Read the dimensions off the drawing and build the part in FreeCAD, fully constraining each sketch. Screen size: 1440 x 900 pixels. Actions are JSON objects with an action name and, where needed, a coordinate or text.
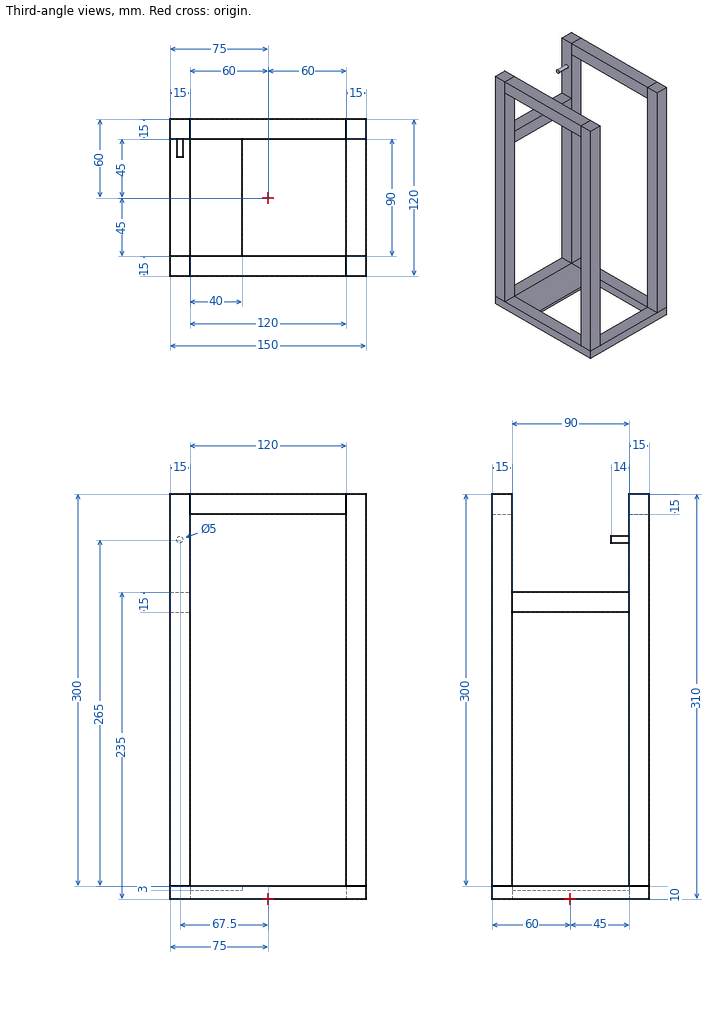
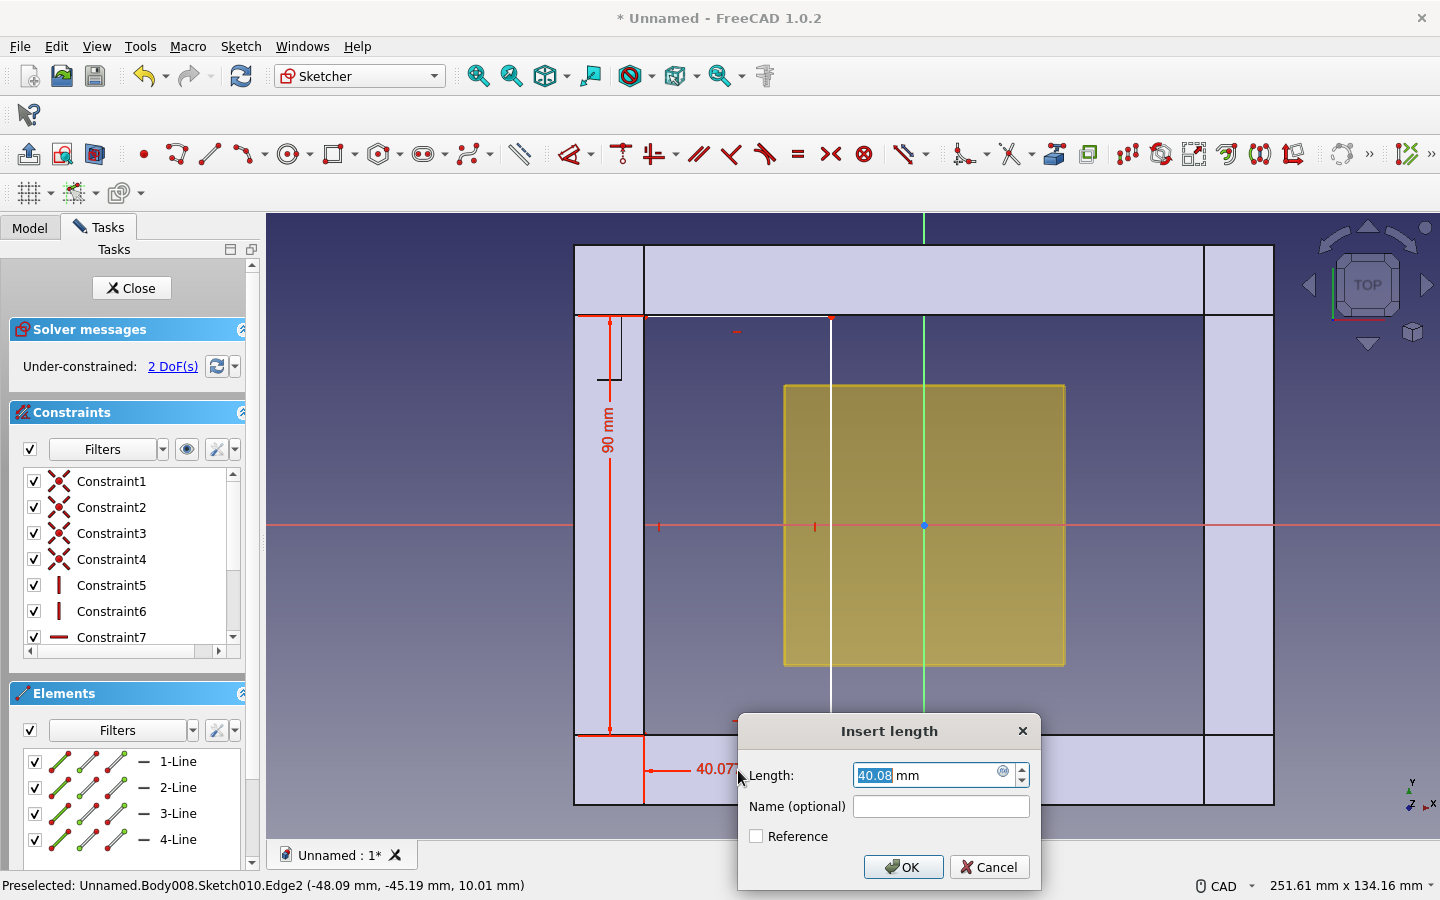
{"action": "type", "text": "40"}
{"action": "key", "text": "Return"}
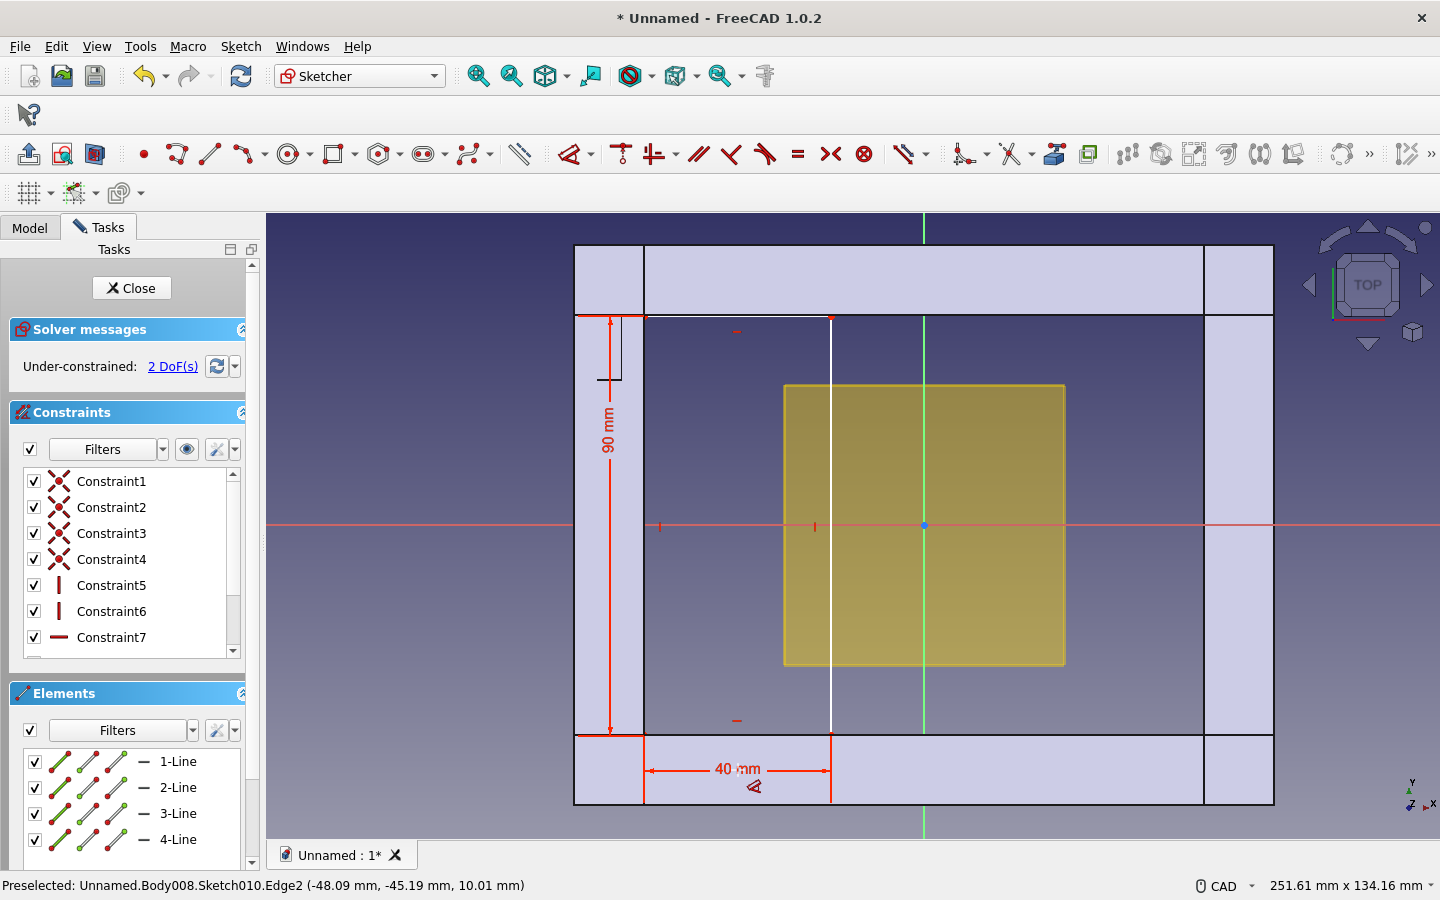
{"action": "left_click", "coordinate": [644, 316]}
{"action": "left_click", "coordinate": [784, 282]}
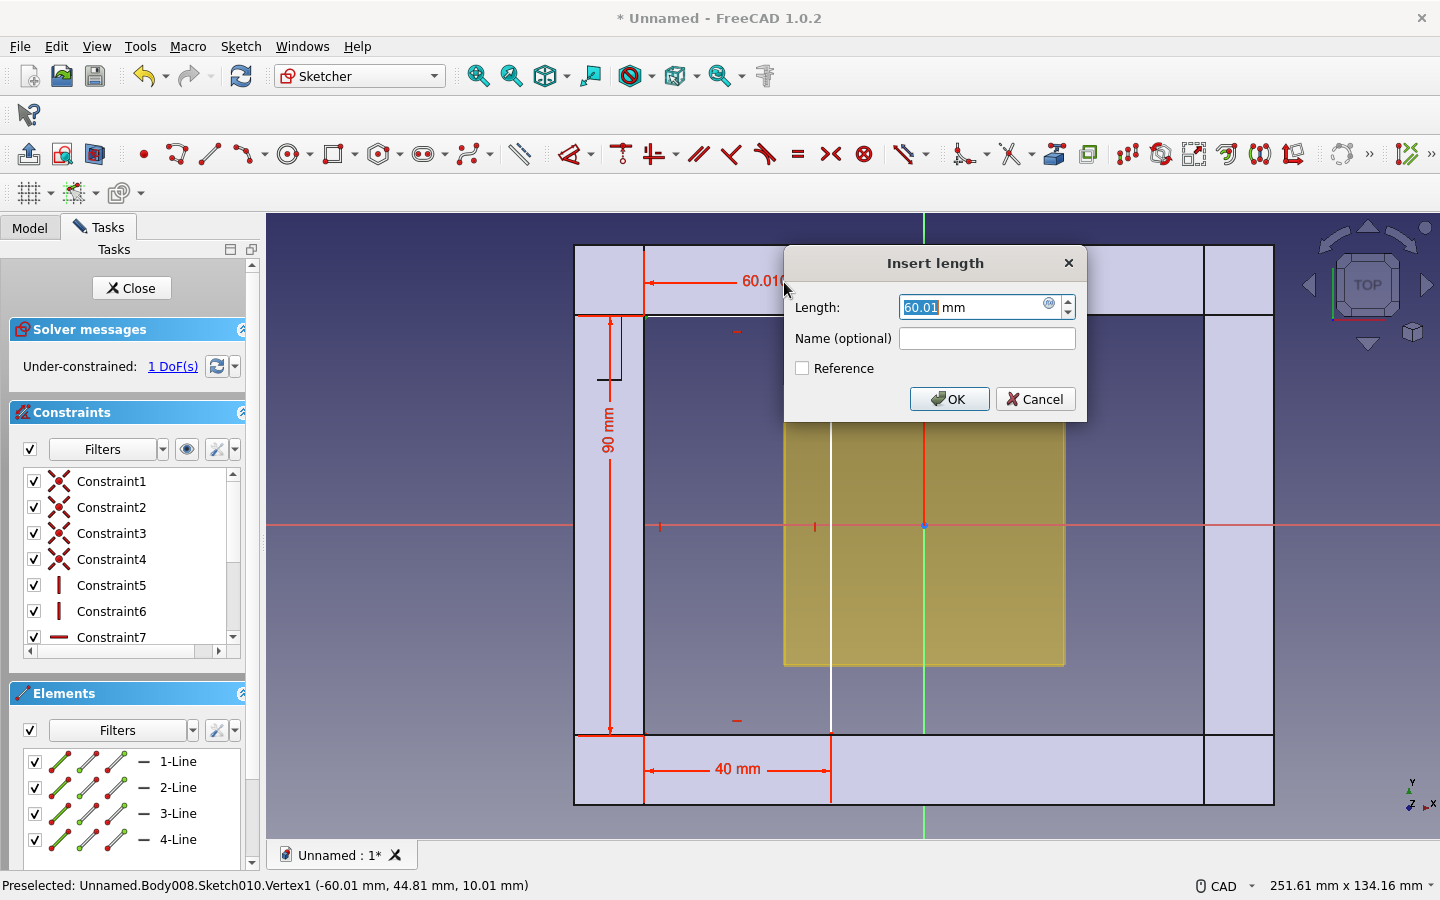
{"action": "type", "text": "60"}
{"action": "key", "text": "Return"}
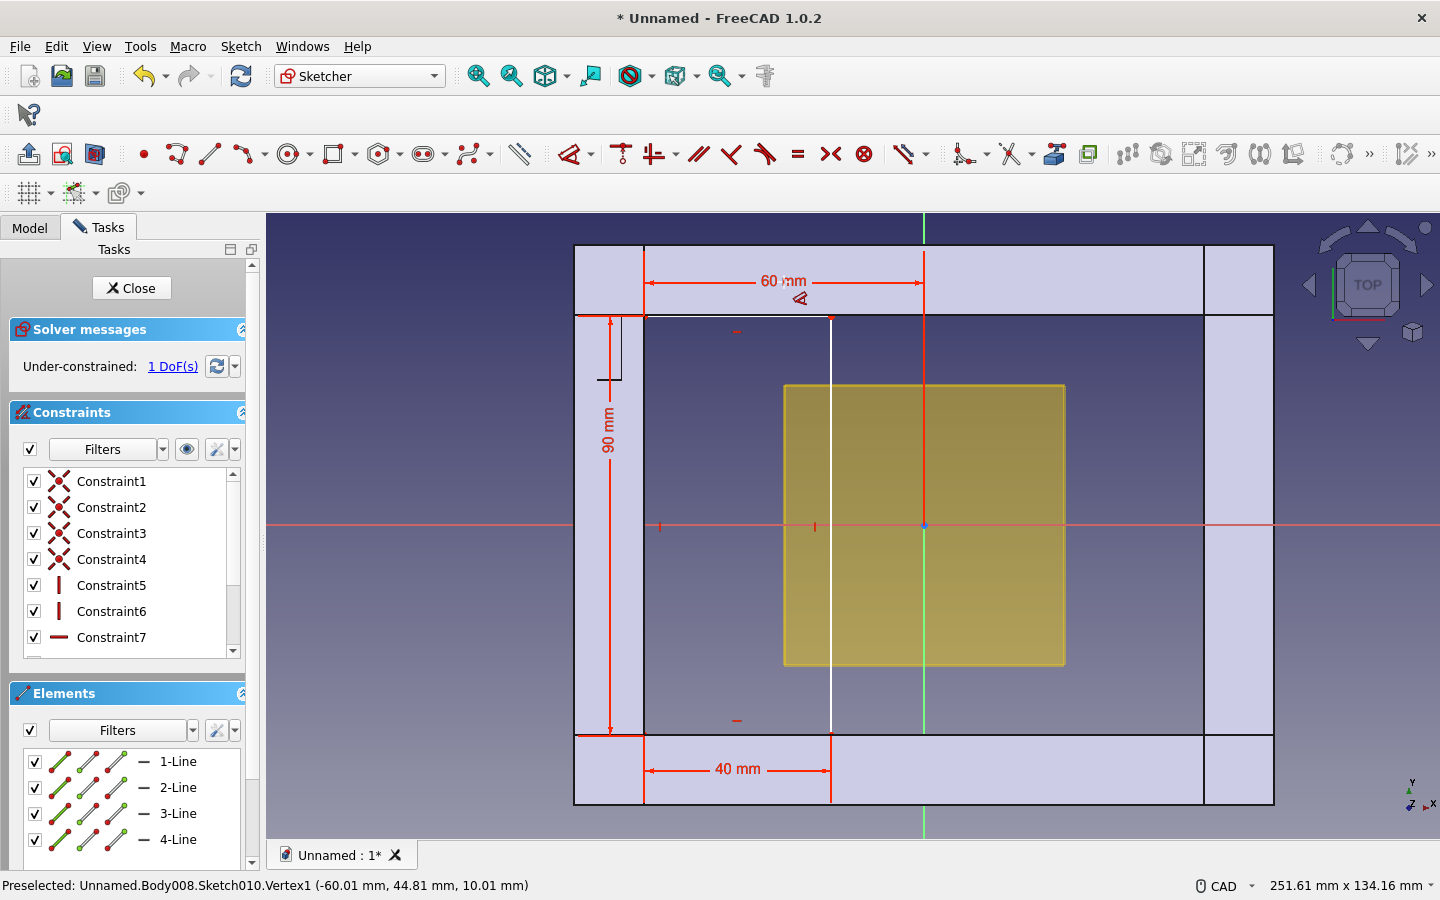
{"action": "left_click", "coordinate": [644, 316]}
{"action": "left_click", "coordinate": [958, 421]}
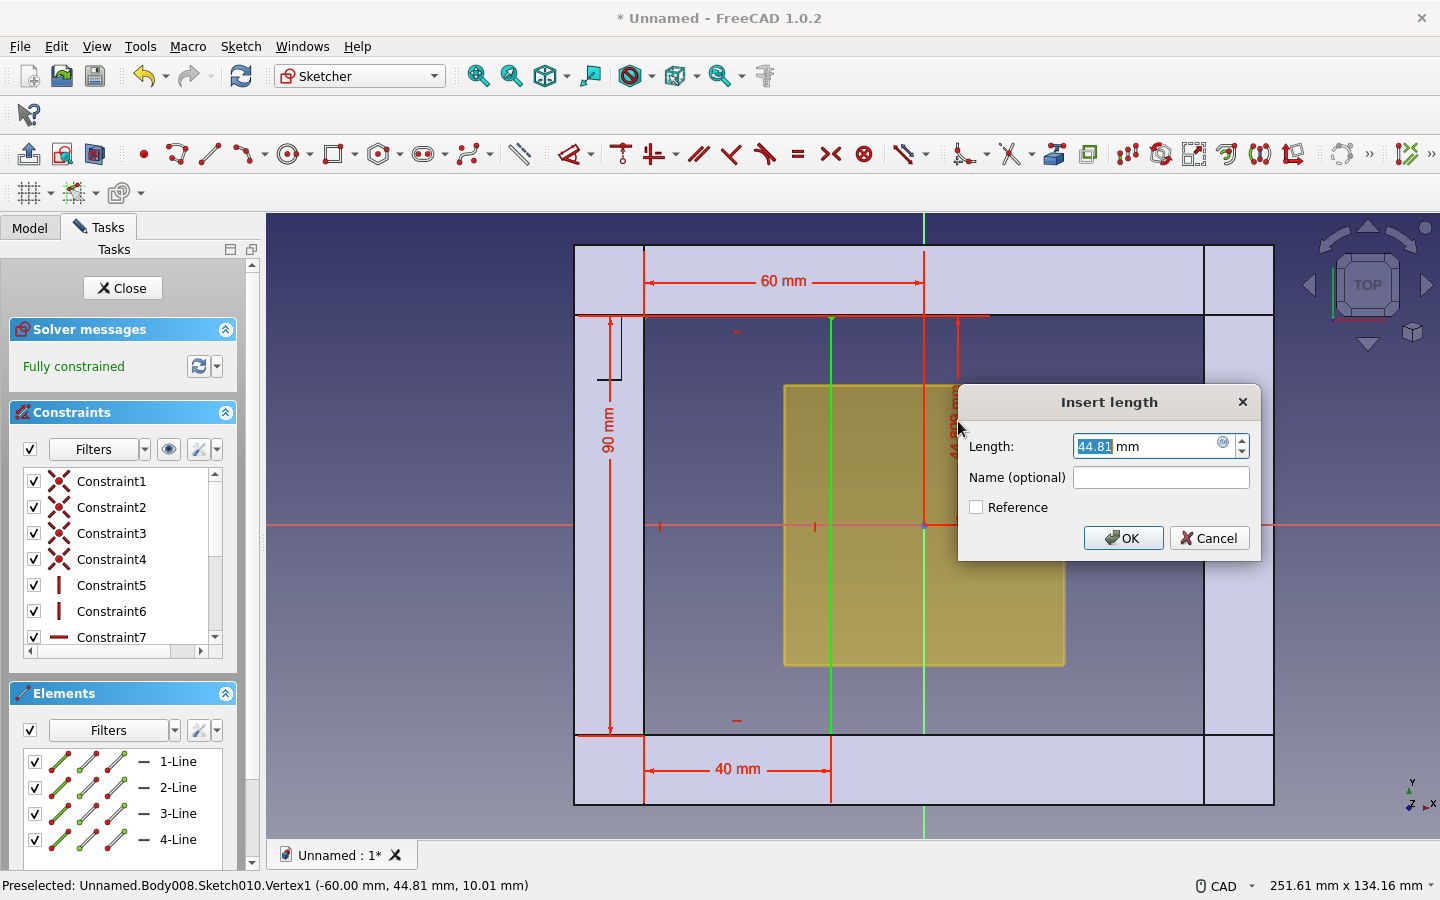
{"action": "type", "text": "45"}
{"action": "key", "text": "Return"}
{"action": "key", "text": "Escape"}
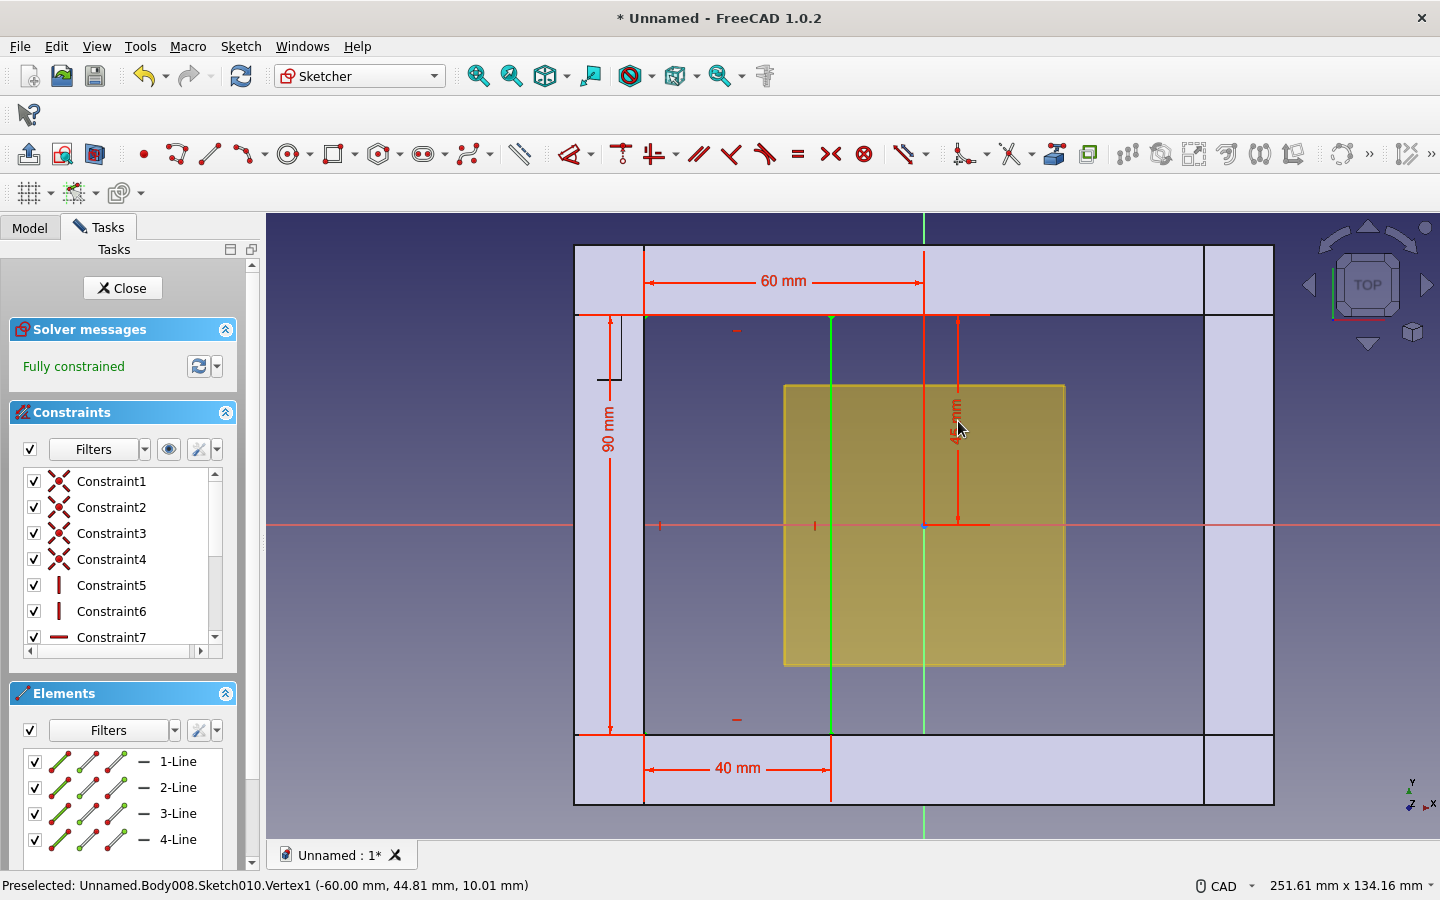
{"action": "left_click", "coordinate": [123, 288]}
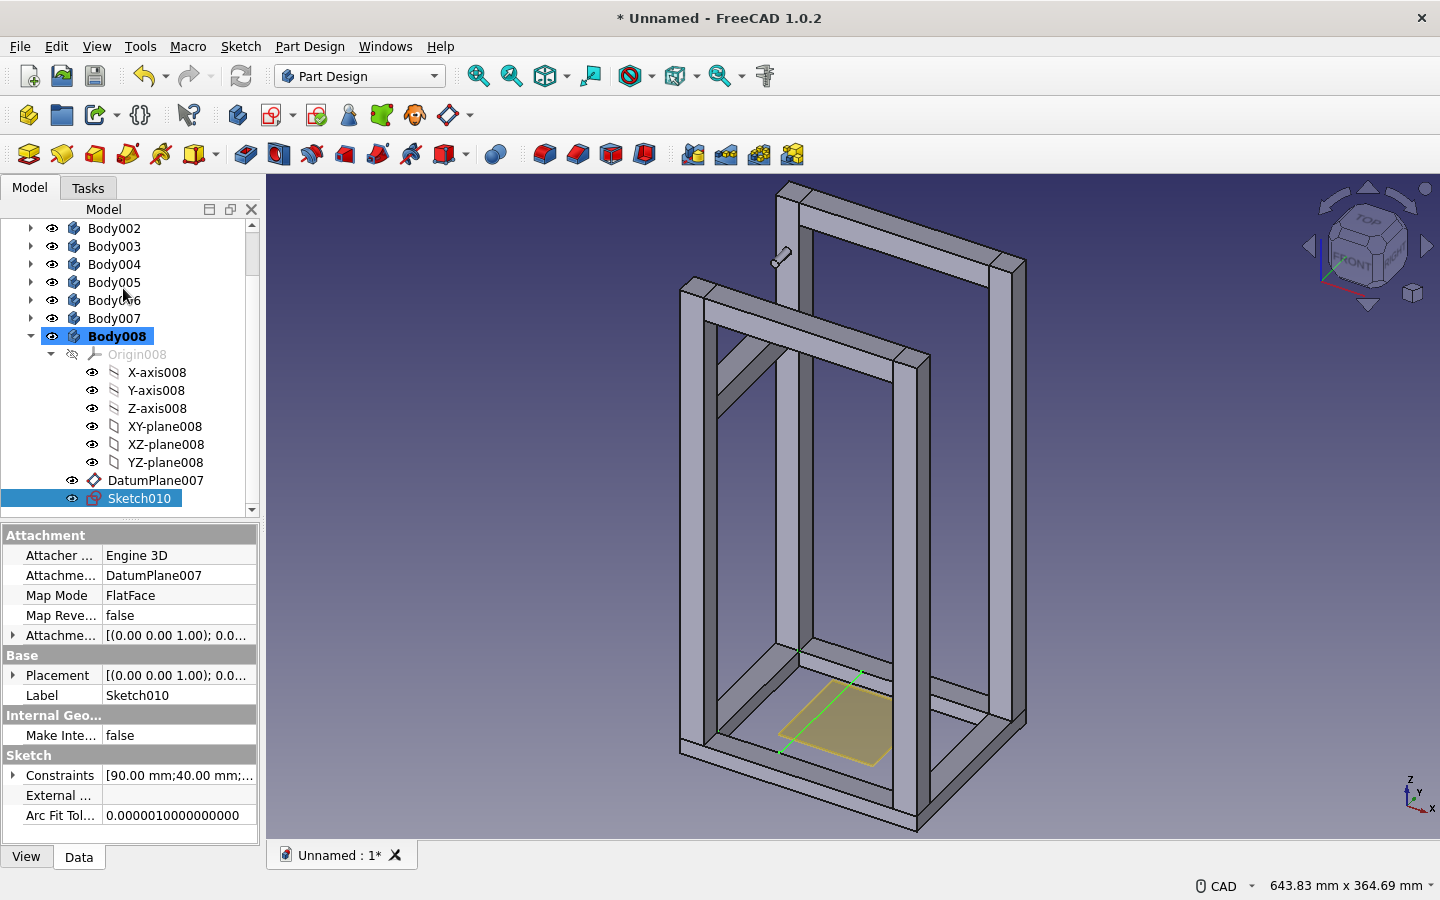
{"action": "left_click", "coordinate": [29, 154]}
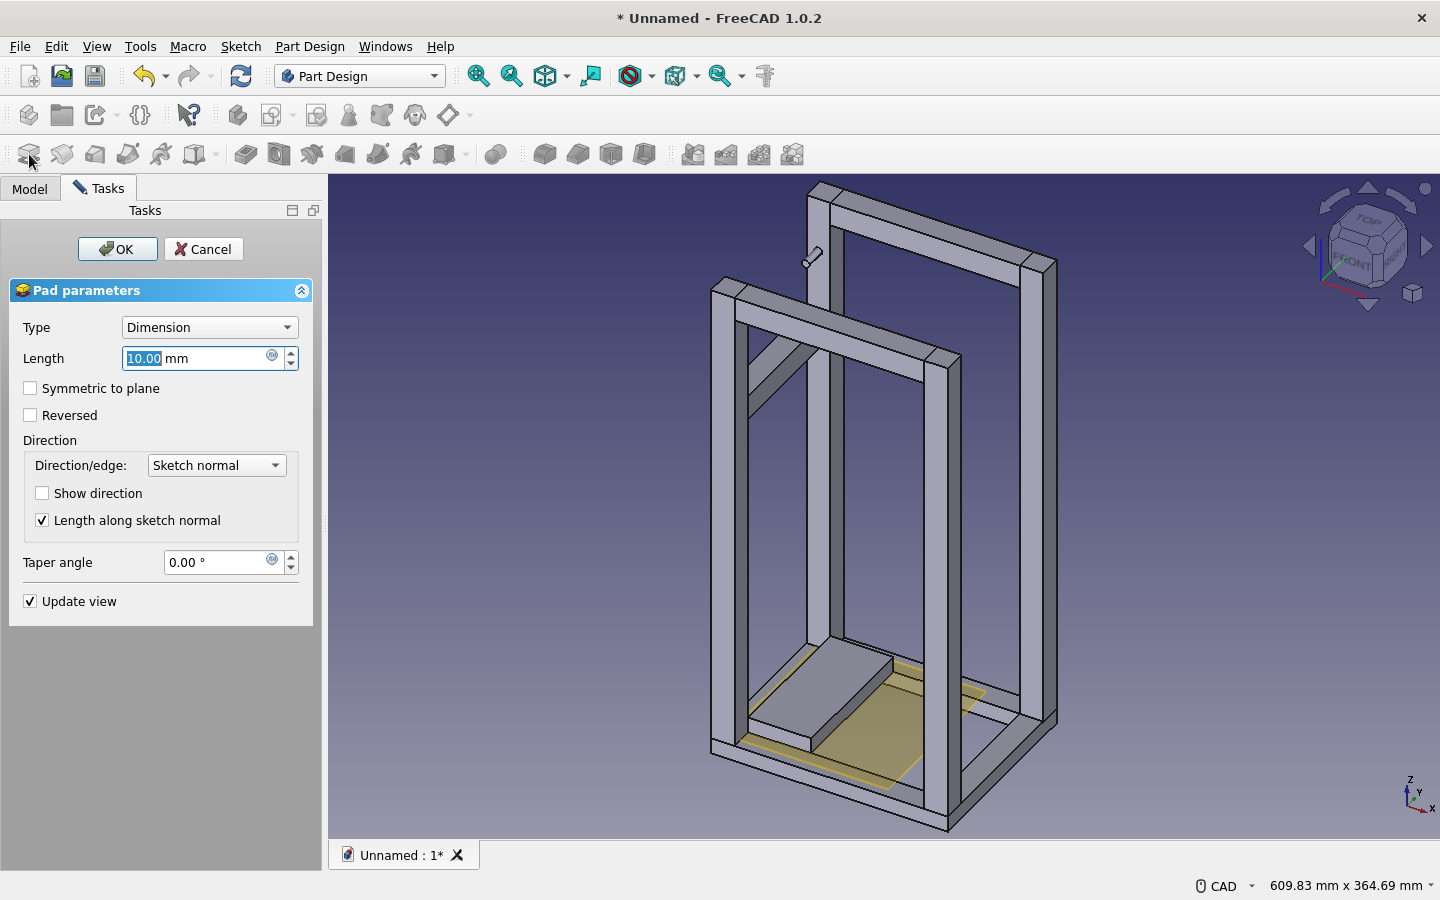
{"action": "type", "text": "3"}
{"action": "key", "text": "Tab"}